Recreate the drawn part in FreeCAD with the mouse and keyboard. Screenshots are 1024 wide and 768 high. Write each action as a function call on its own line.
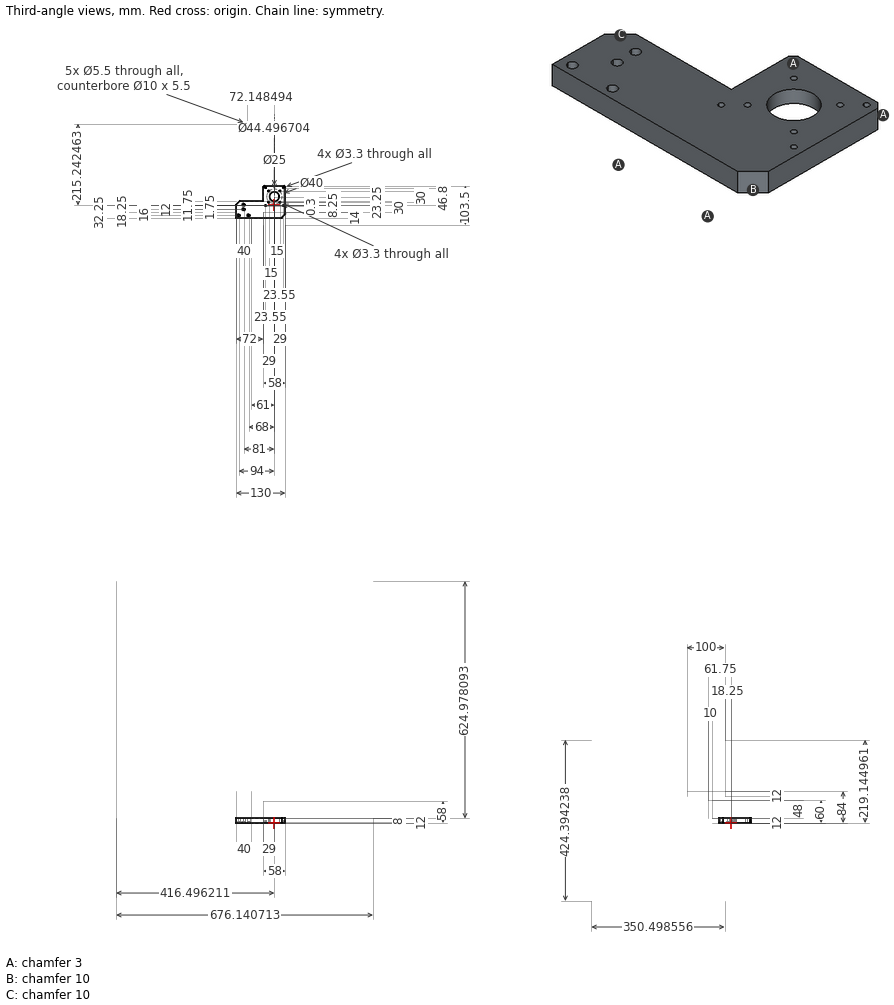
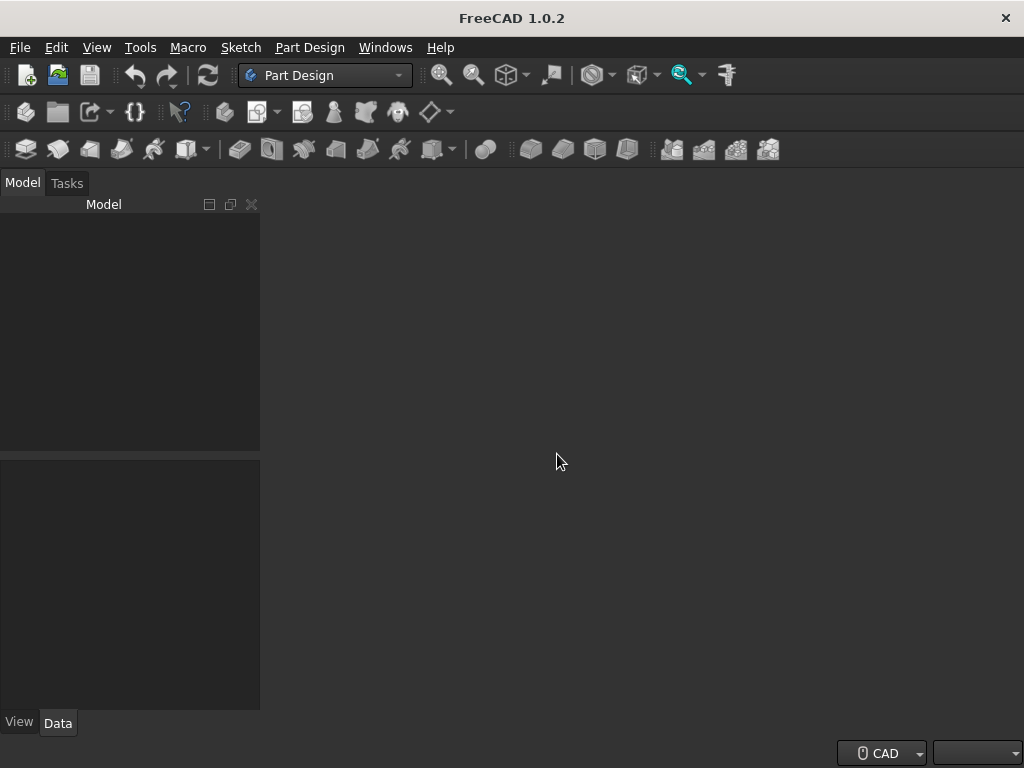
click(26, 76)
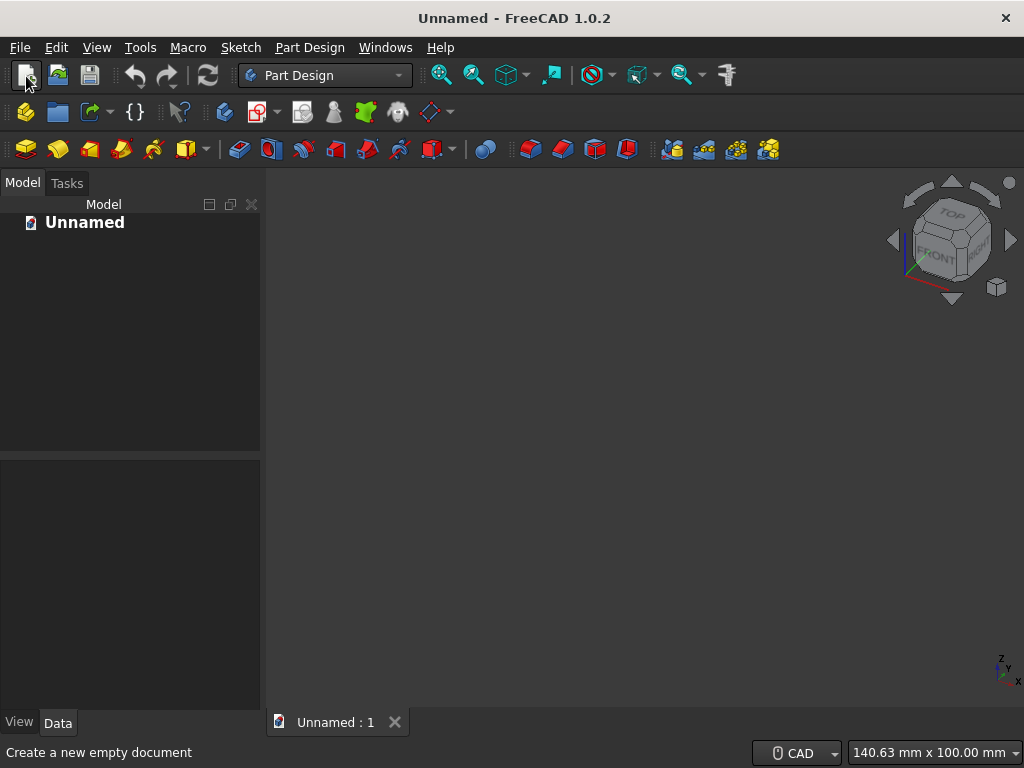
click(258, 112)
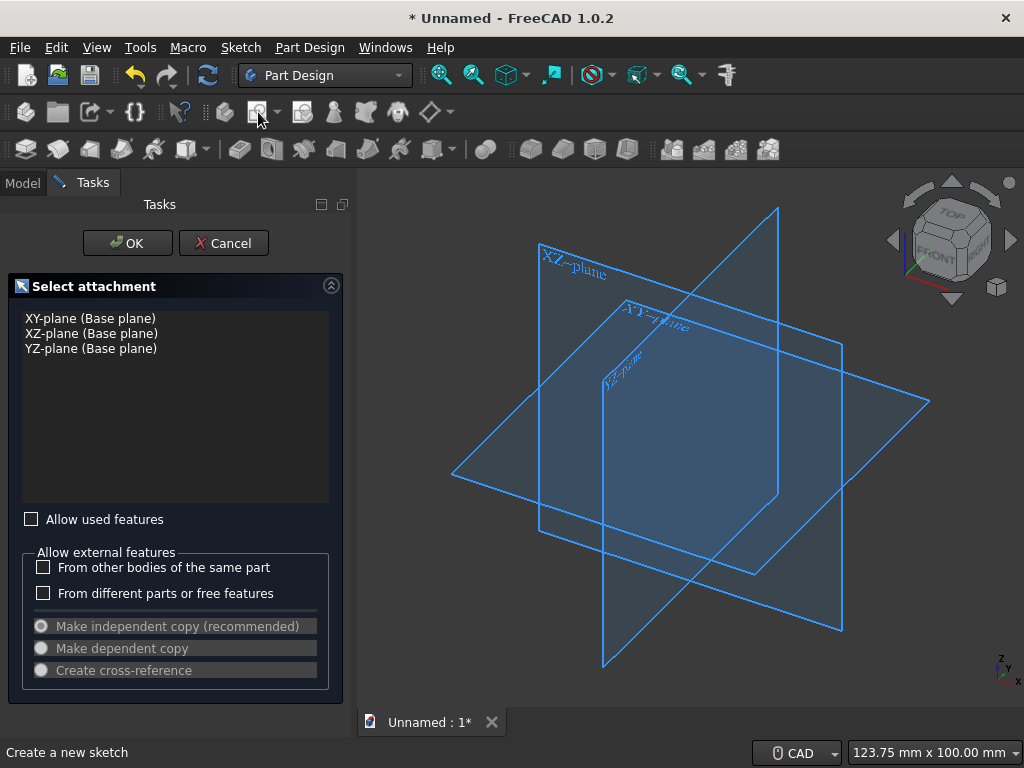
click(82, 318)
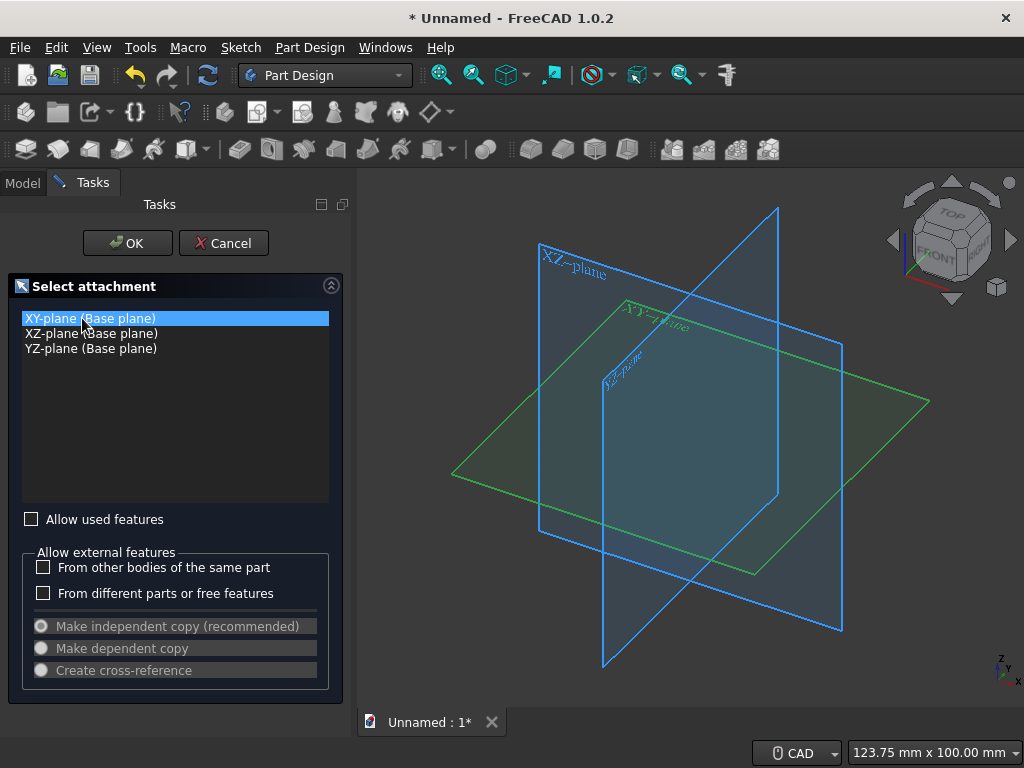
click(128, 243)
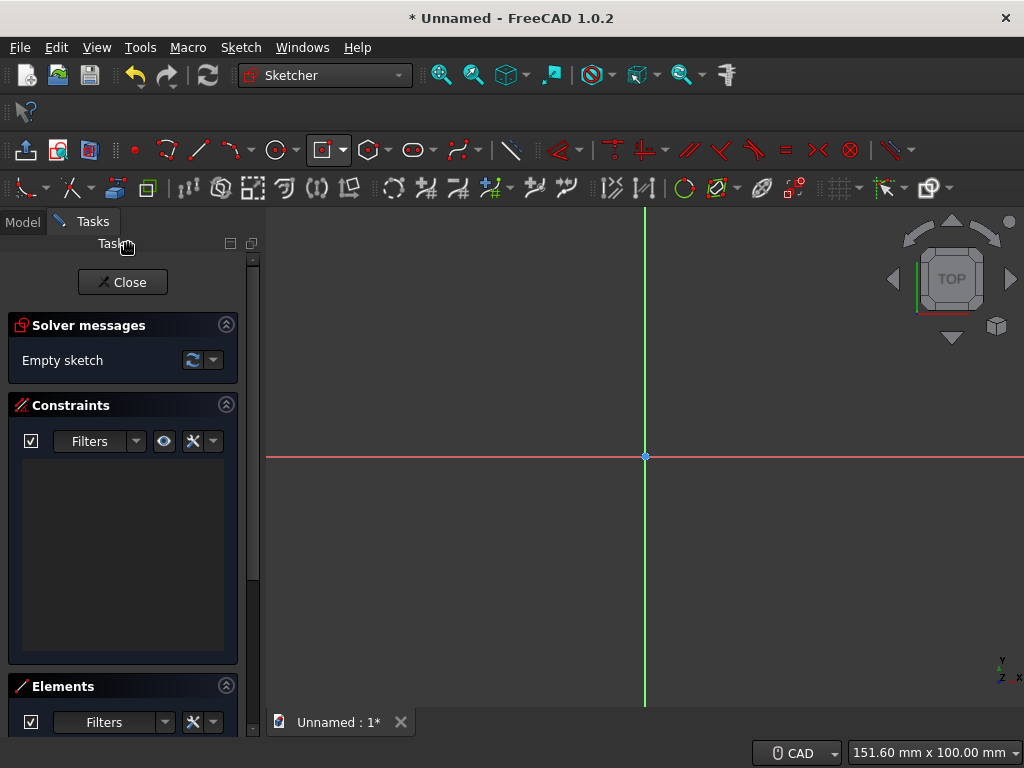
scroll(493, 457, down, 3)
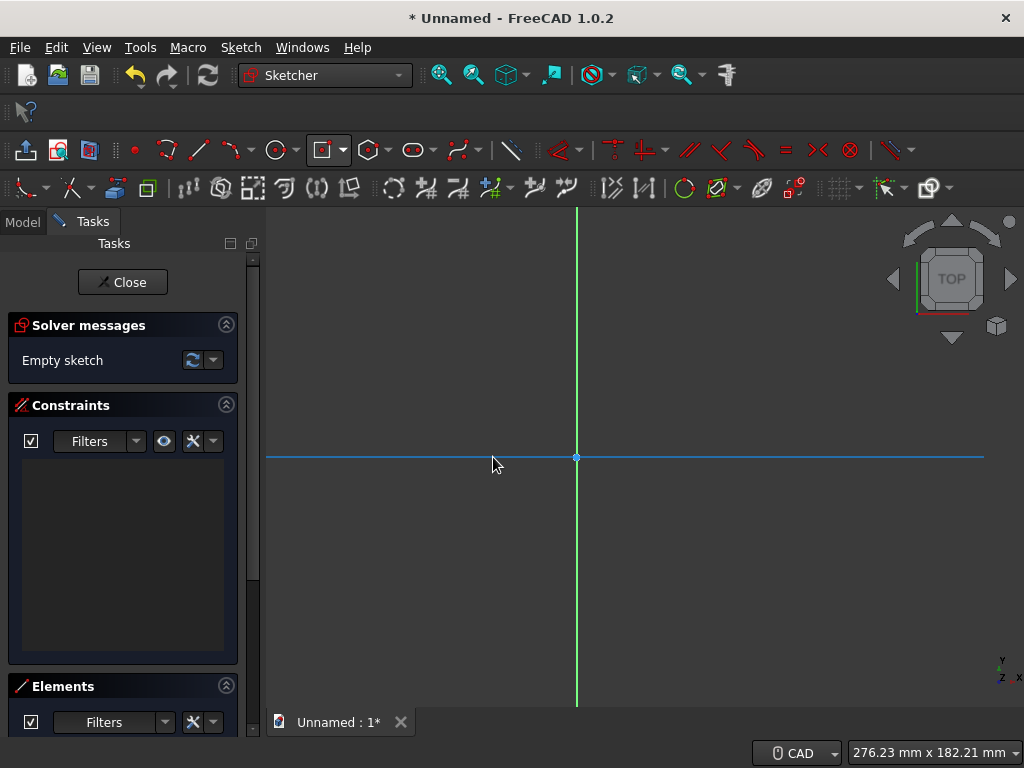
click(322, 150)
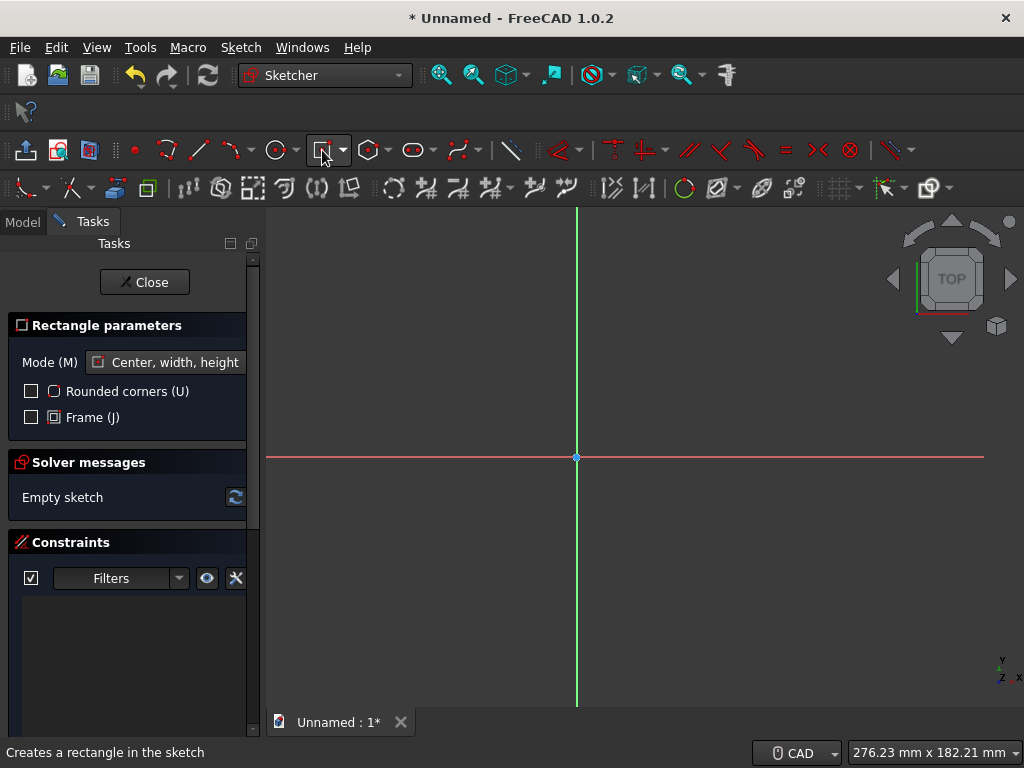
click(577, 457)
move(656, 315)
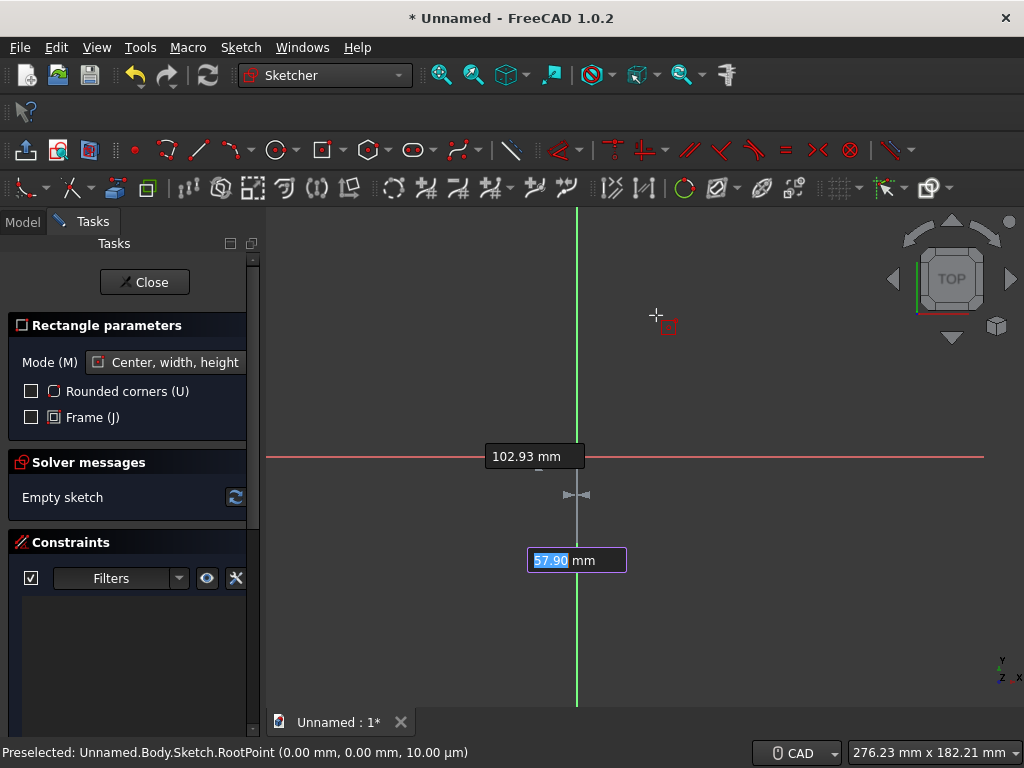
text(58)
key(Tab)
text(103.5)
key(Return)
key(Escape)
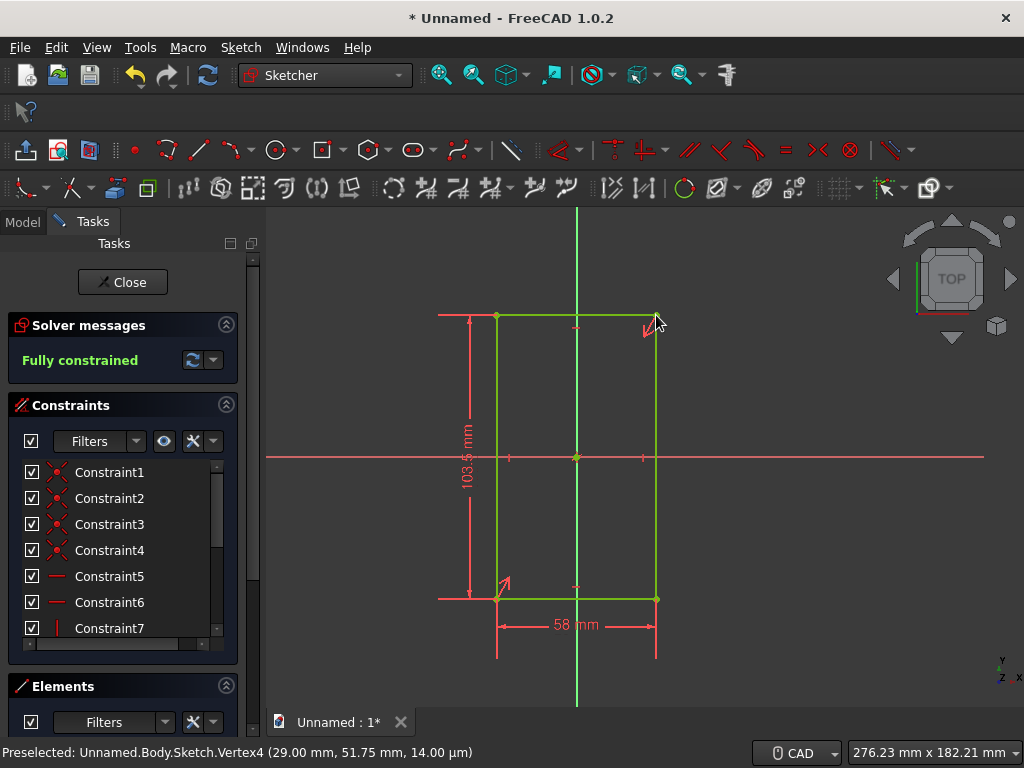
click(123, 282)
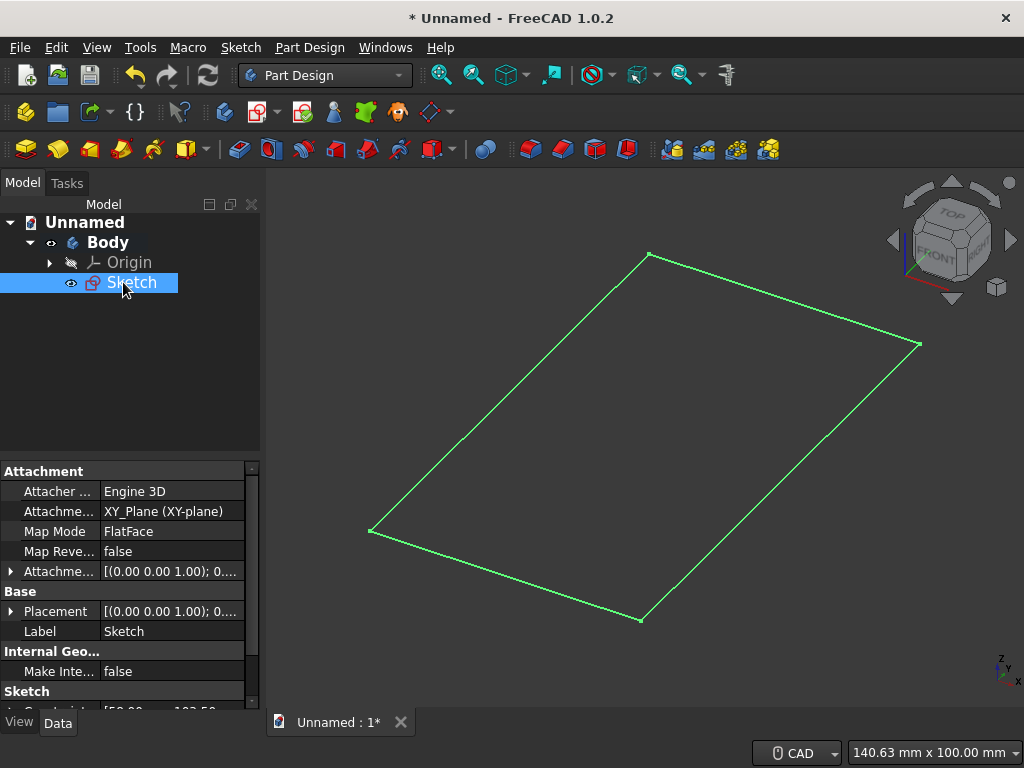
click(26, 150)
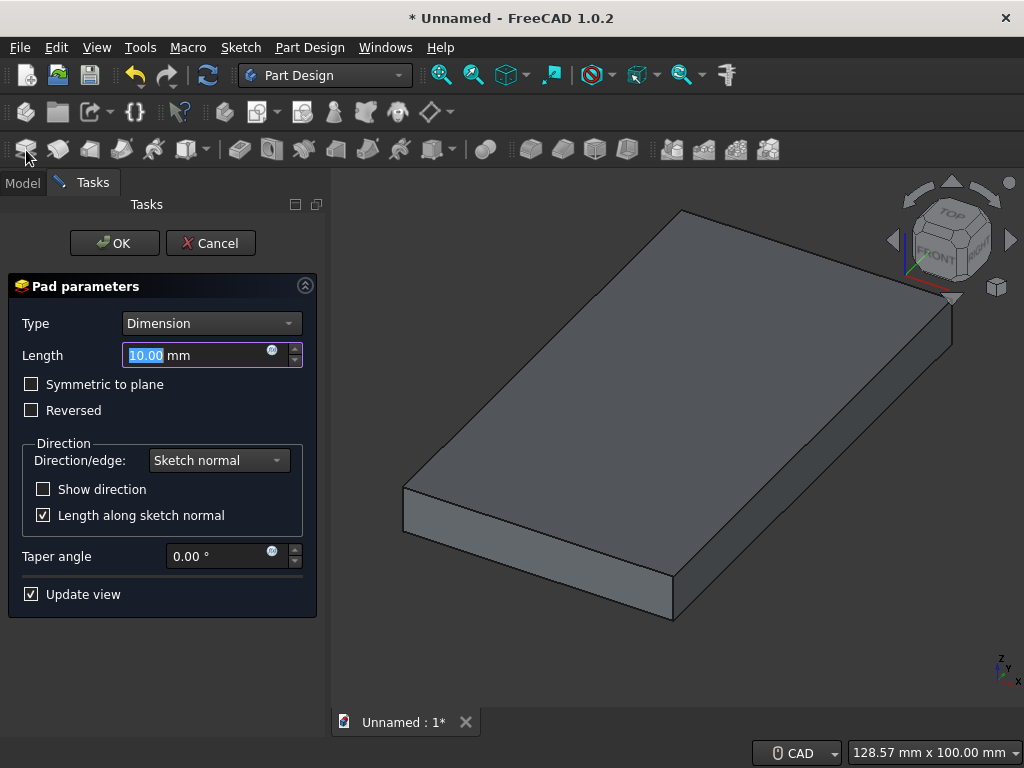
text(12)
key(Tab)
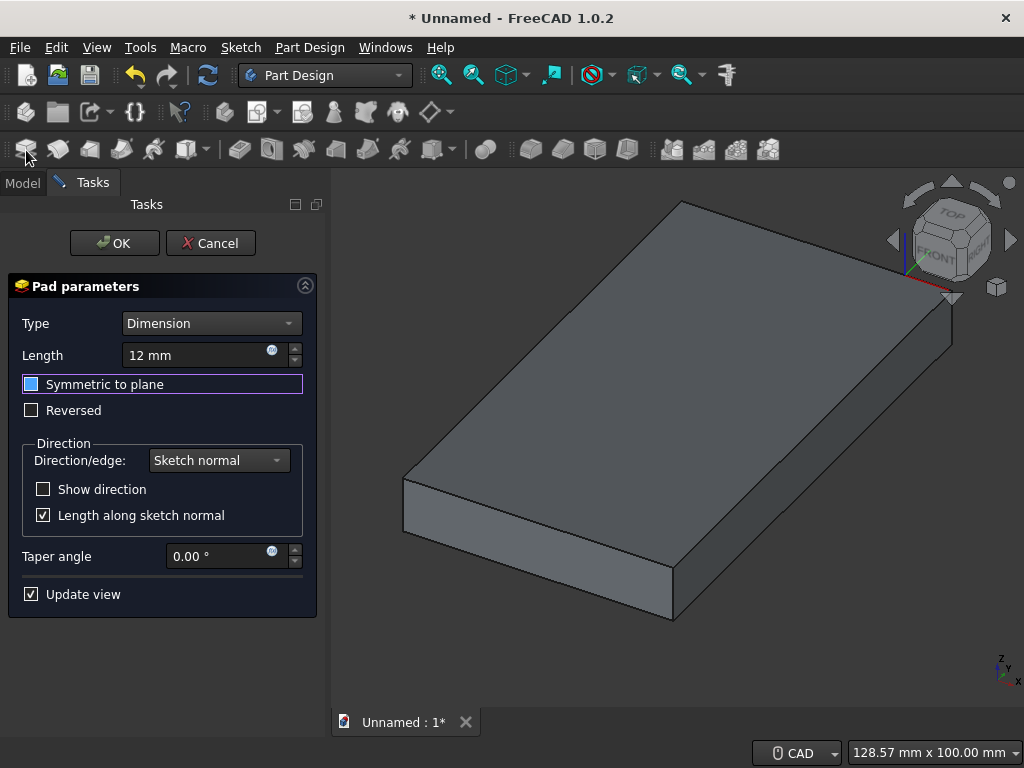
click(115, 243)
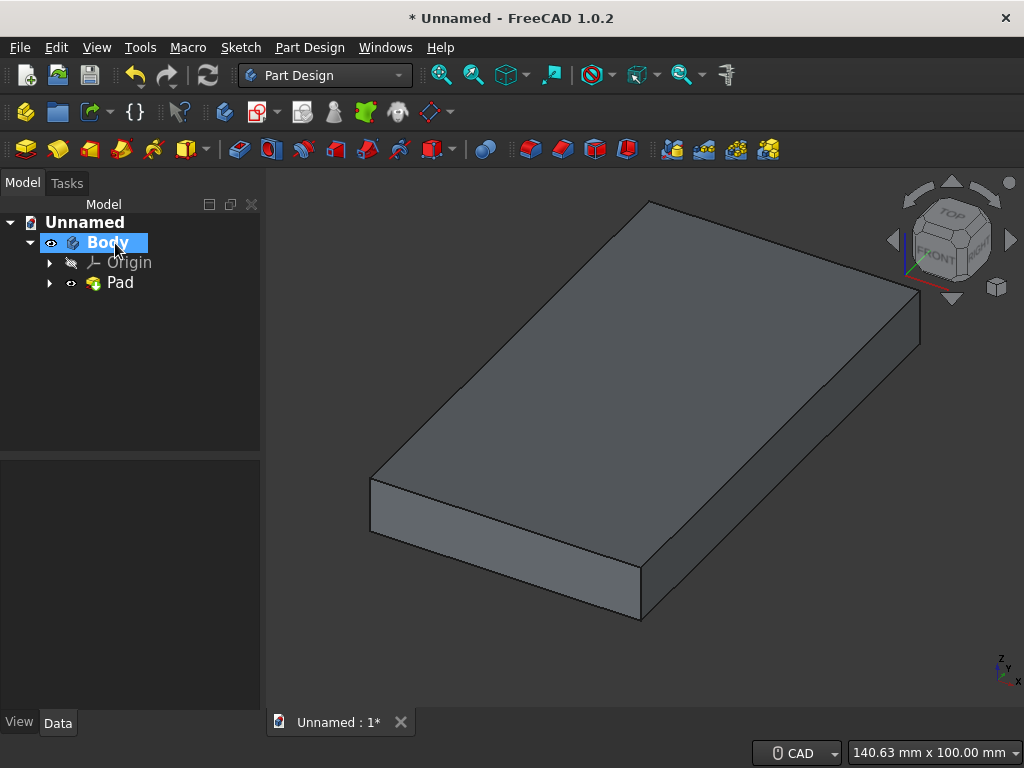
click(258, 112)